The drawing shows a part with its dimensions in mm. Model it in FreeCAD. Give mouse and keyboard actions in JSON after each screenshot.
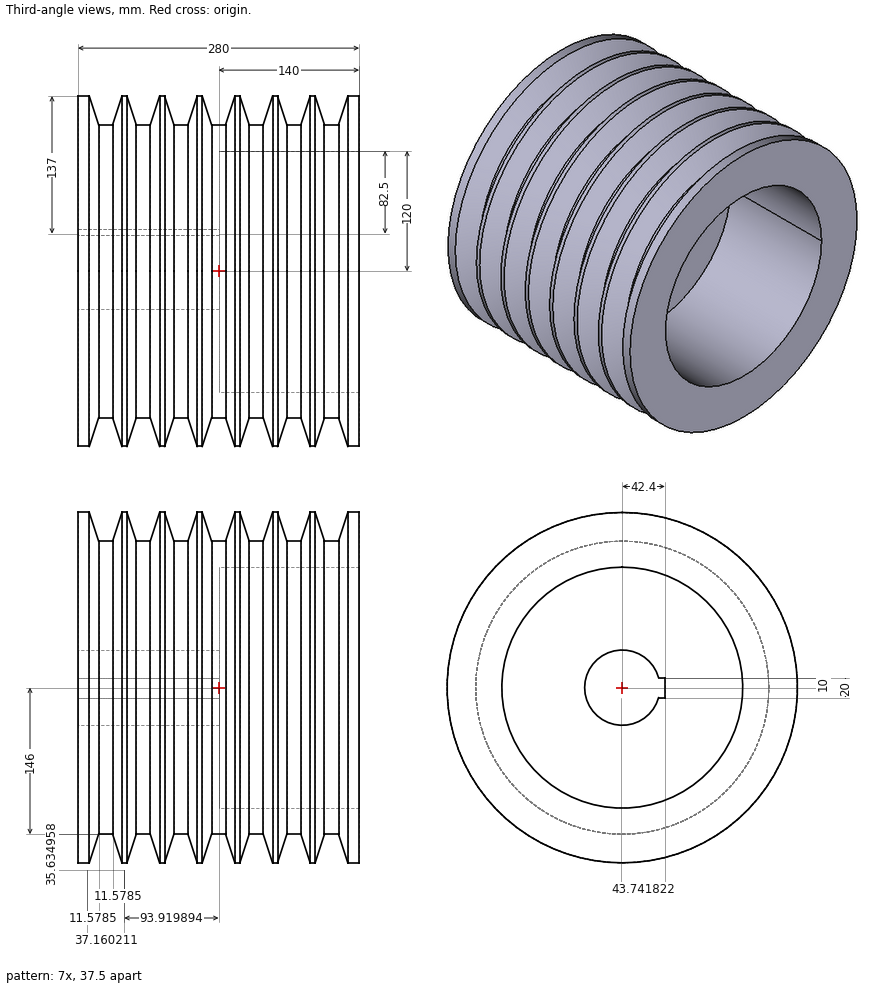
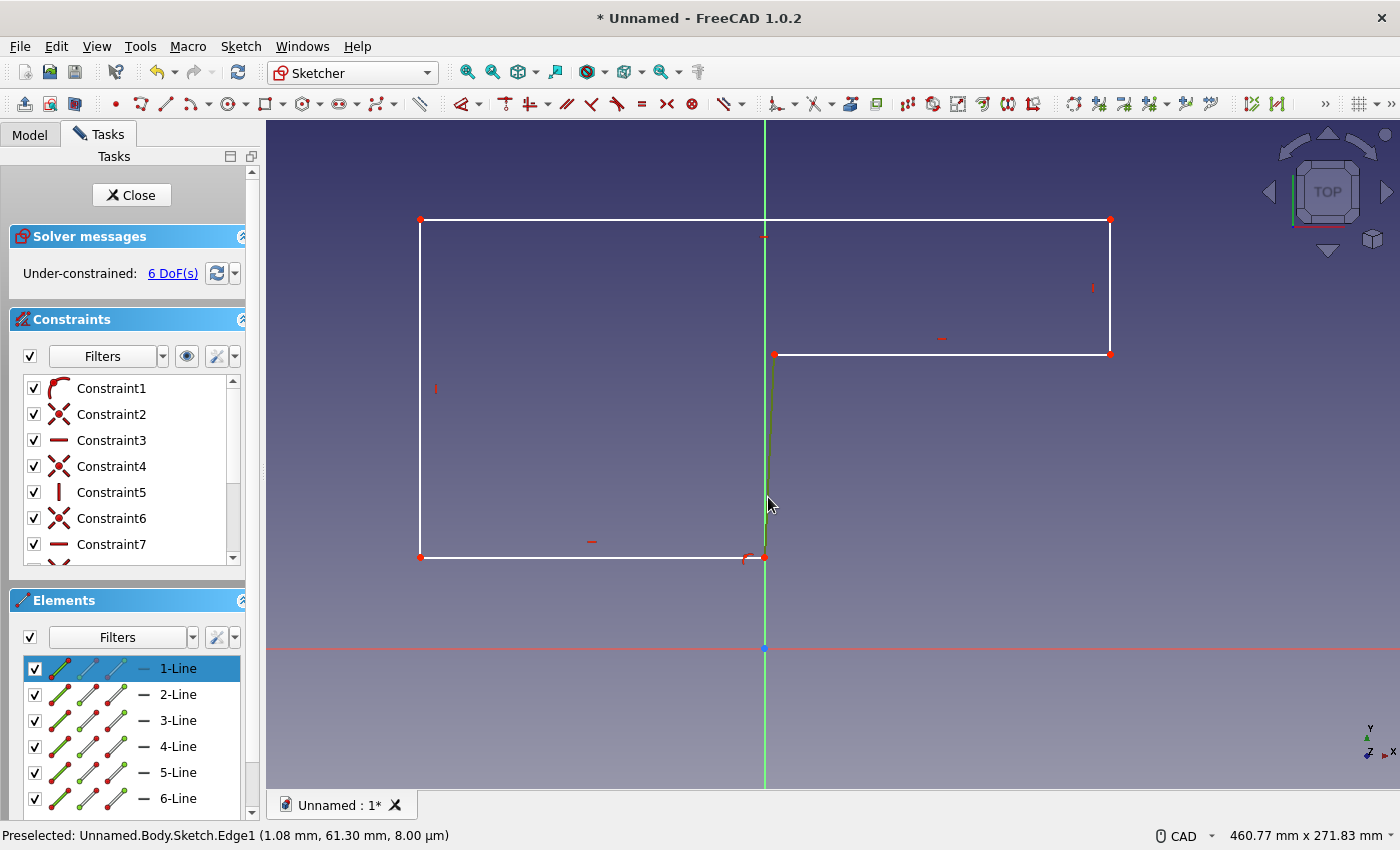
{"action": "key", "text": "v"}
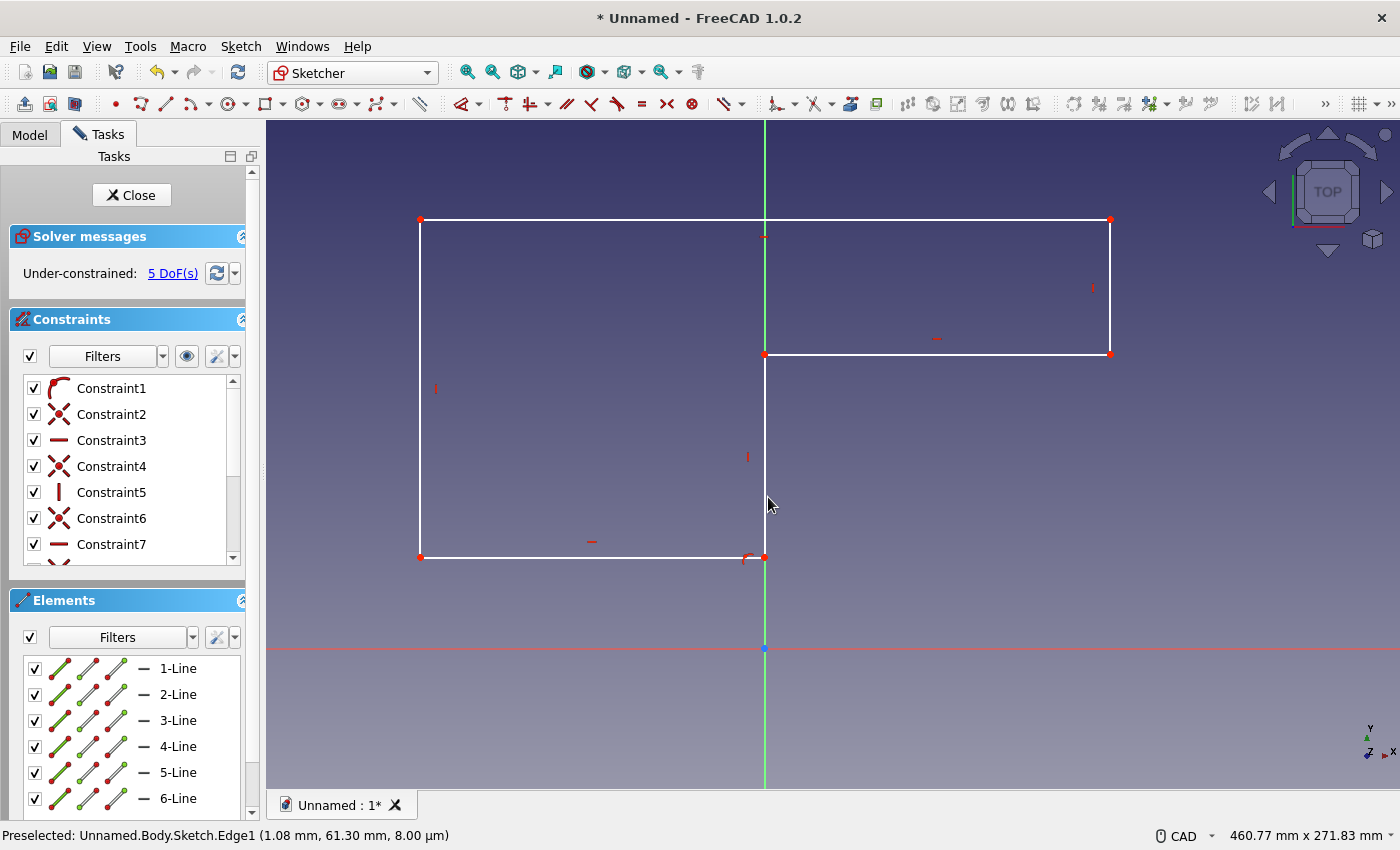
{"action": "left_click", "coordinate": [868, 355]}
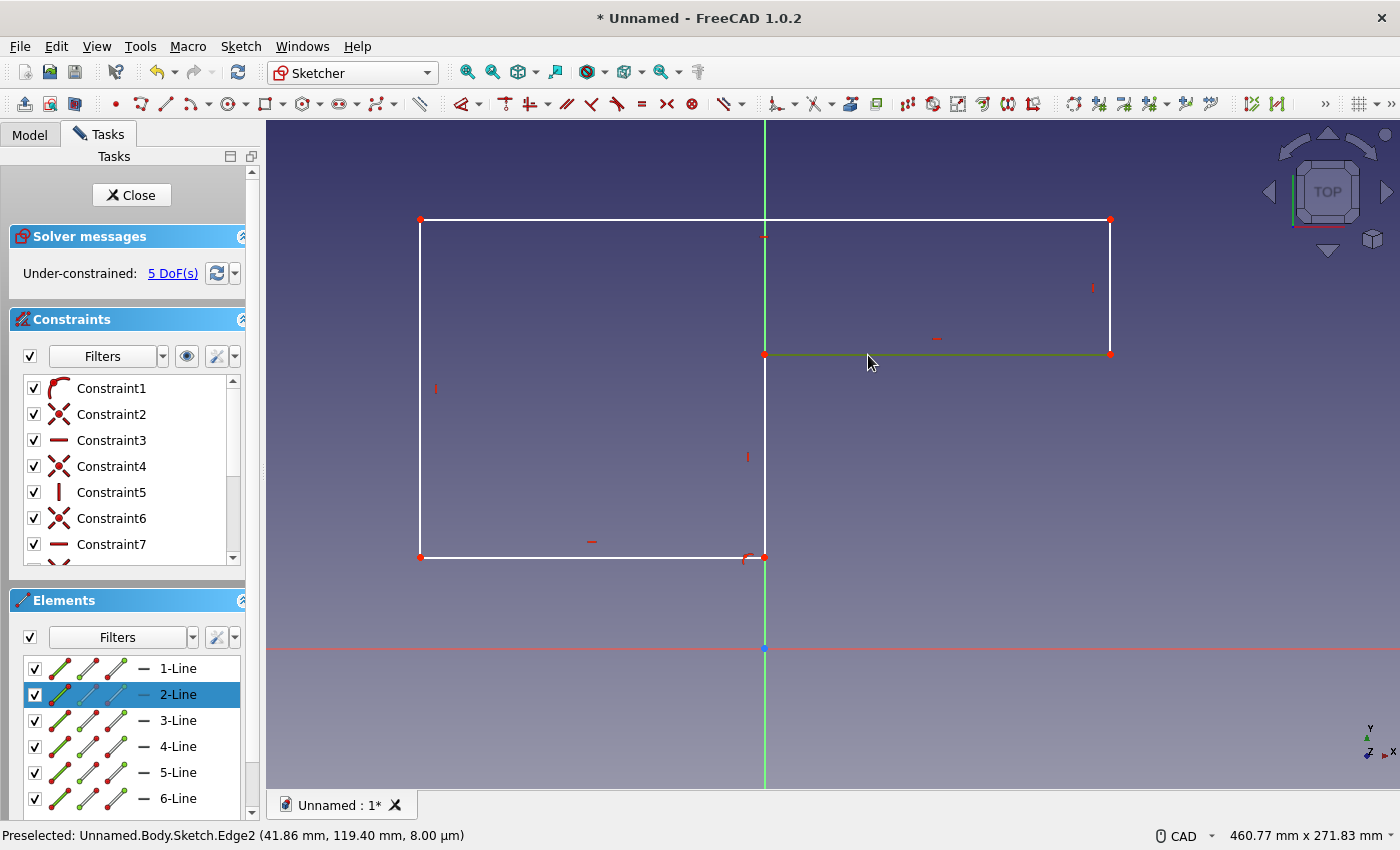
{"action": "left_click", "coordinate": [478, 104]}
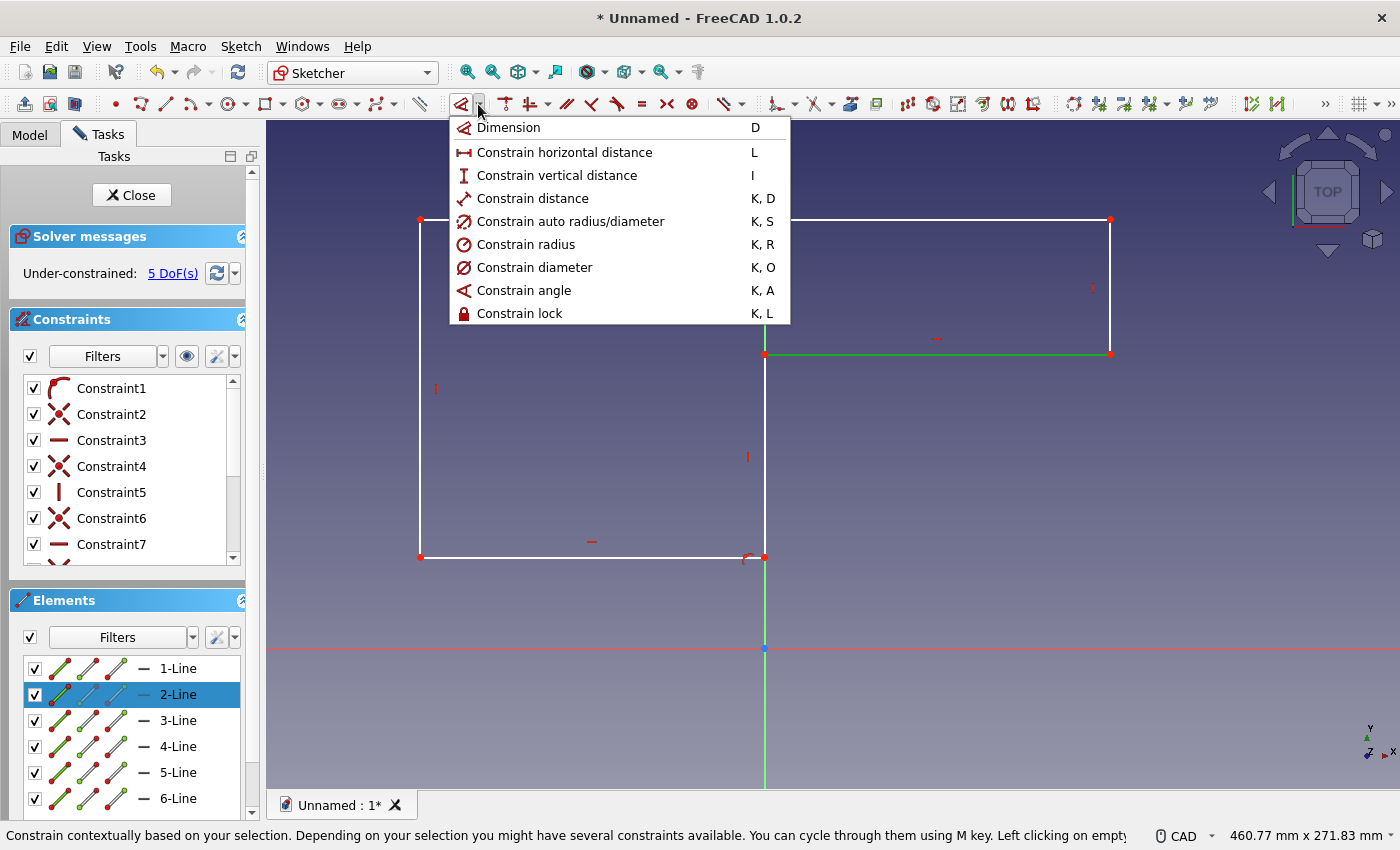
{"action": "left_click", "coordinate": [620, 152]}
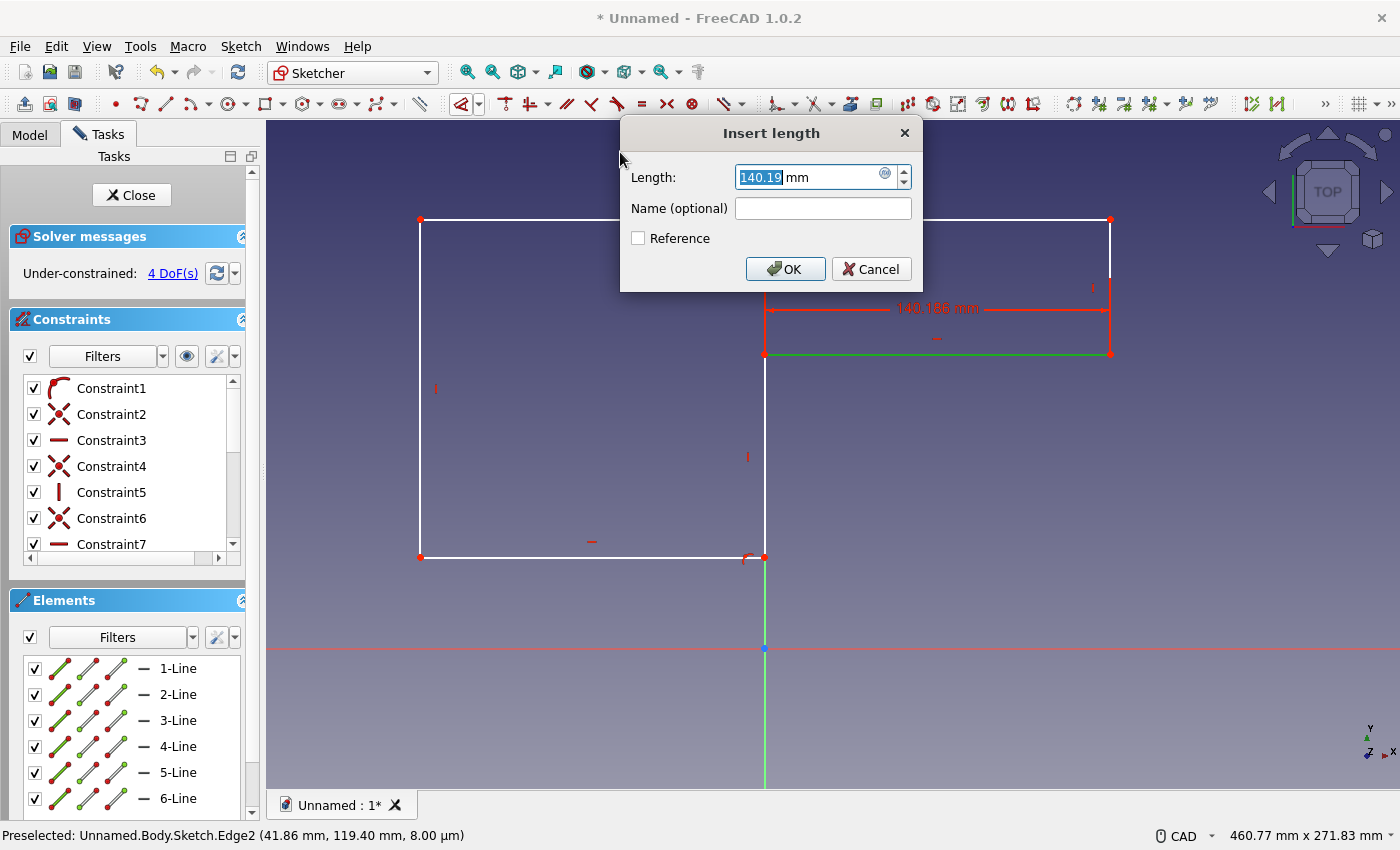
{"action": "type", "text": "140"}
{"action": "key", "text": "Return"}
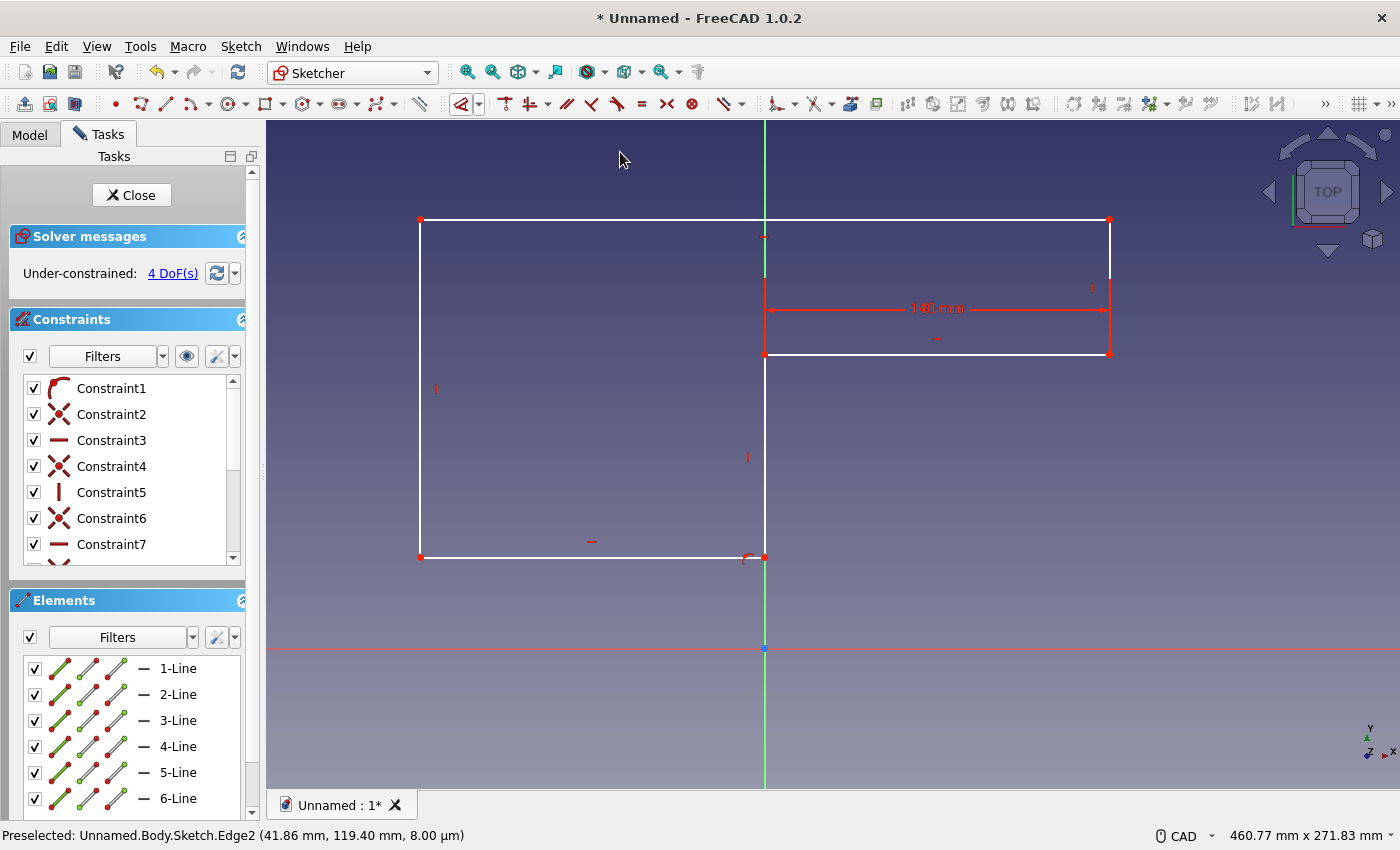
{"action": "left_click", "coordinate": [903, 220]}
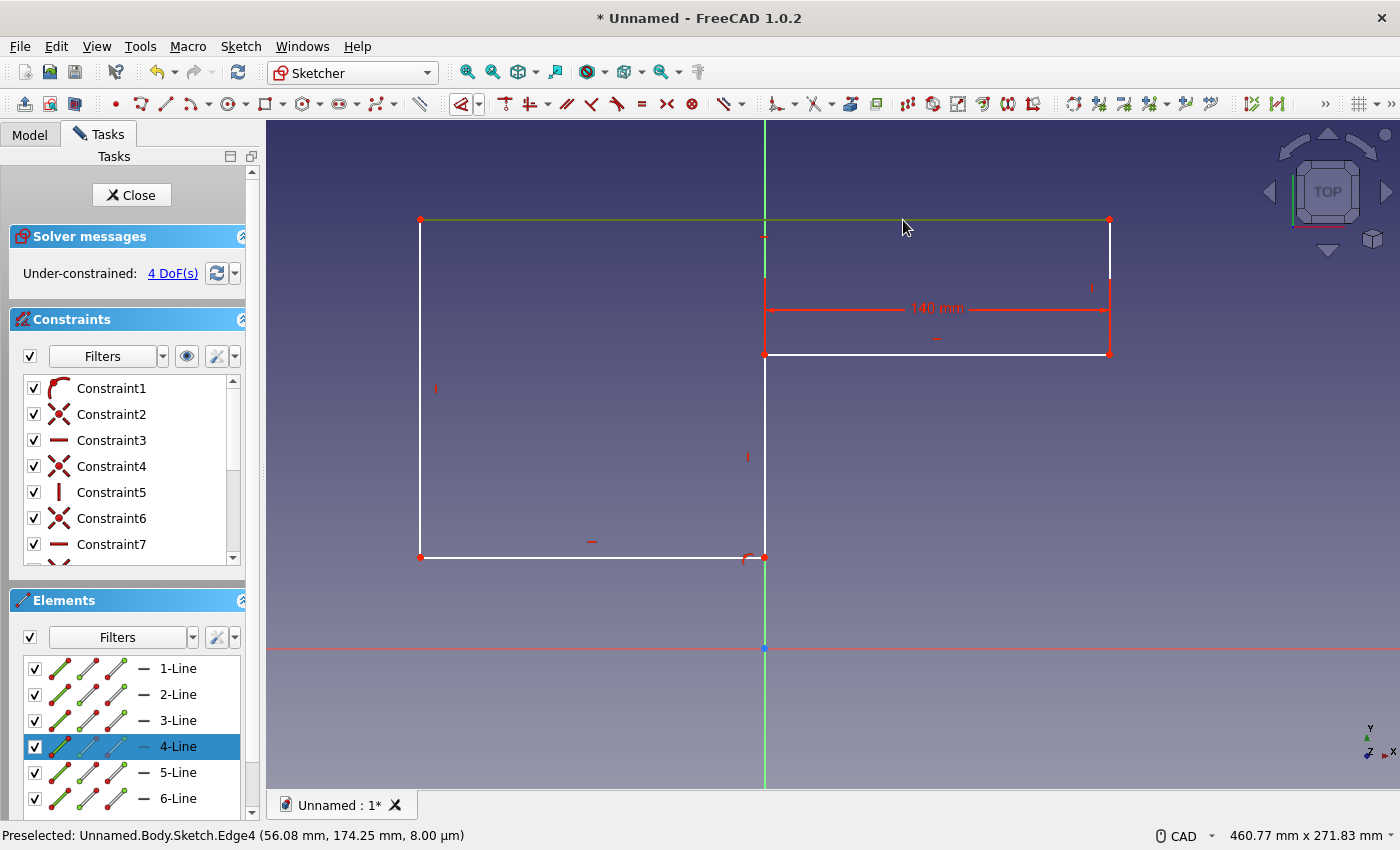
{"action": "left_click", "coordinate": [478, 104]}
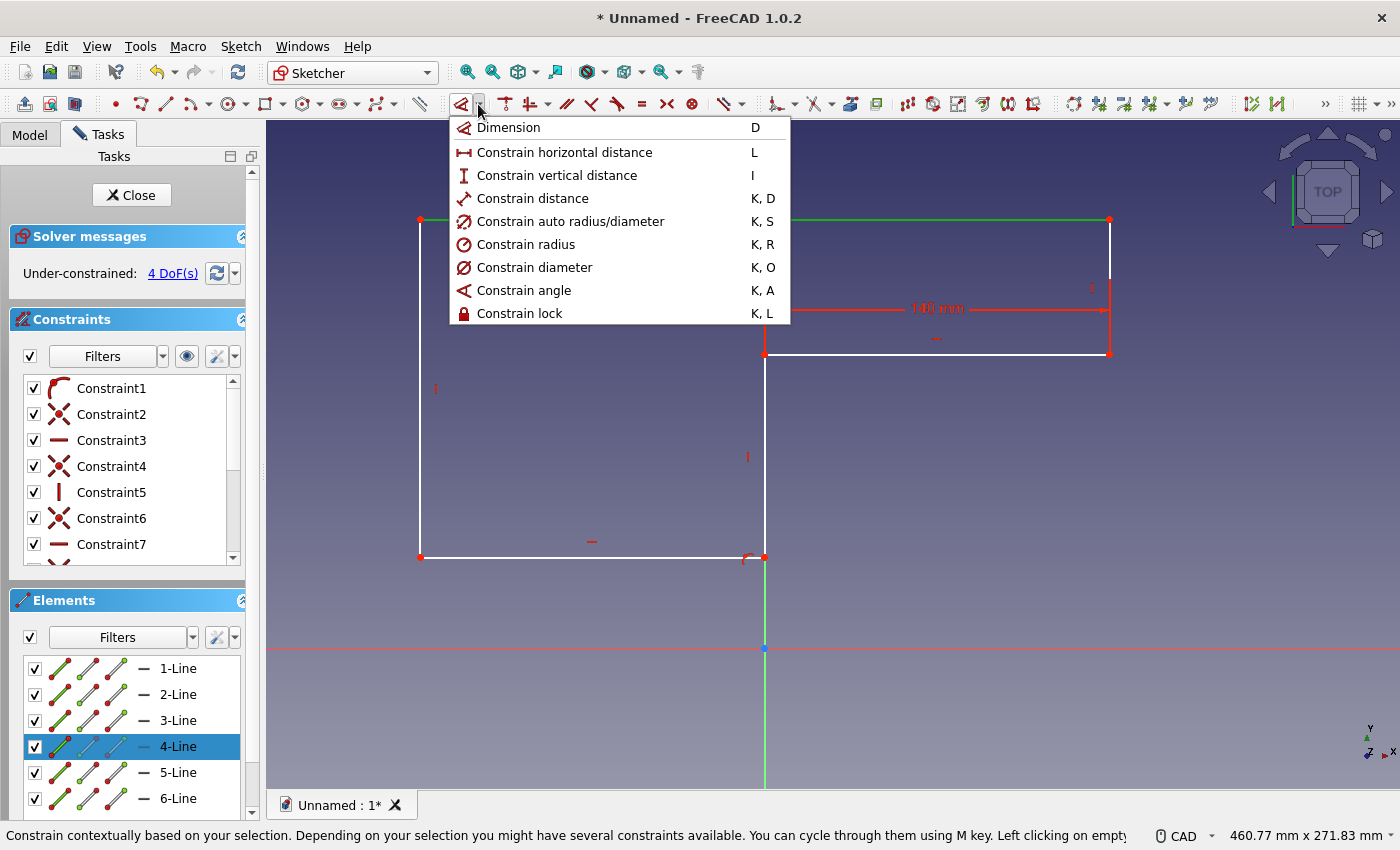
{"action": "left_click", "coordinate": [620, 152]}